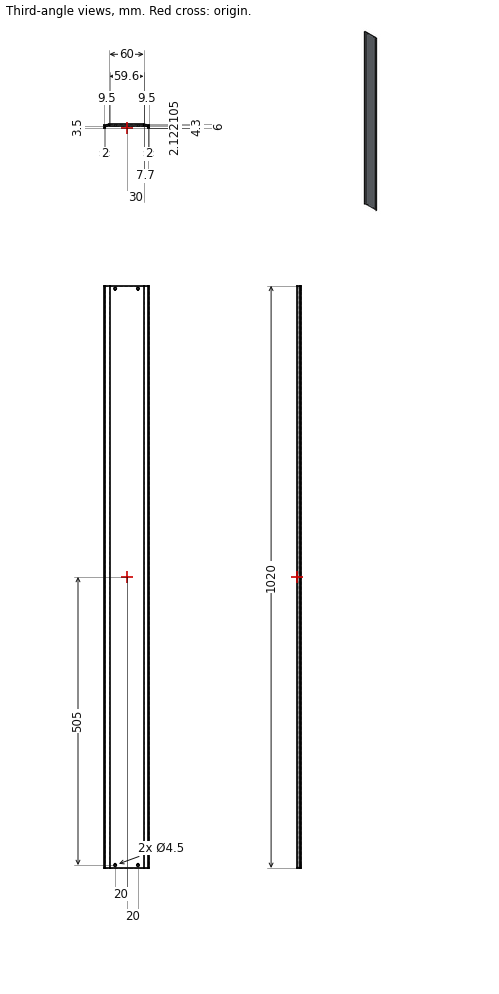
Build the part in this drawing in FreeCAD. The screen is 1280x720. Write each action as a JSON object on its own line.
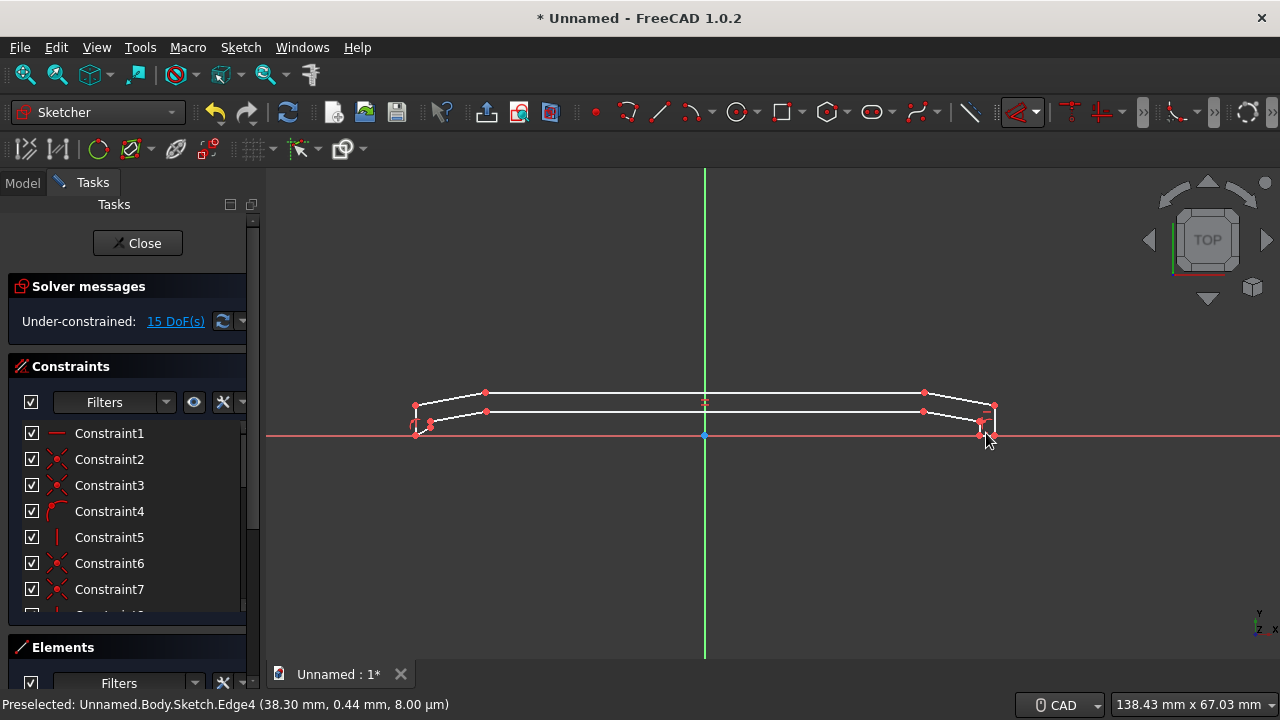
{"action": "scroll", "coordinate": [426, 430], "scroll_direction": "up", "scroll_amount": 5}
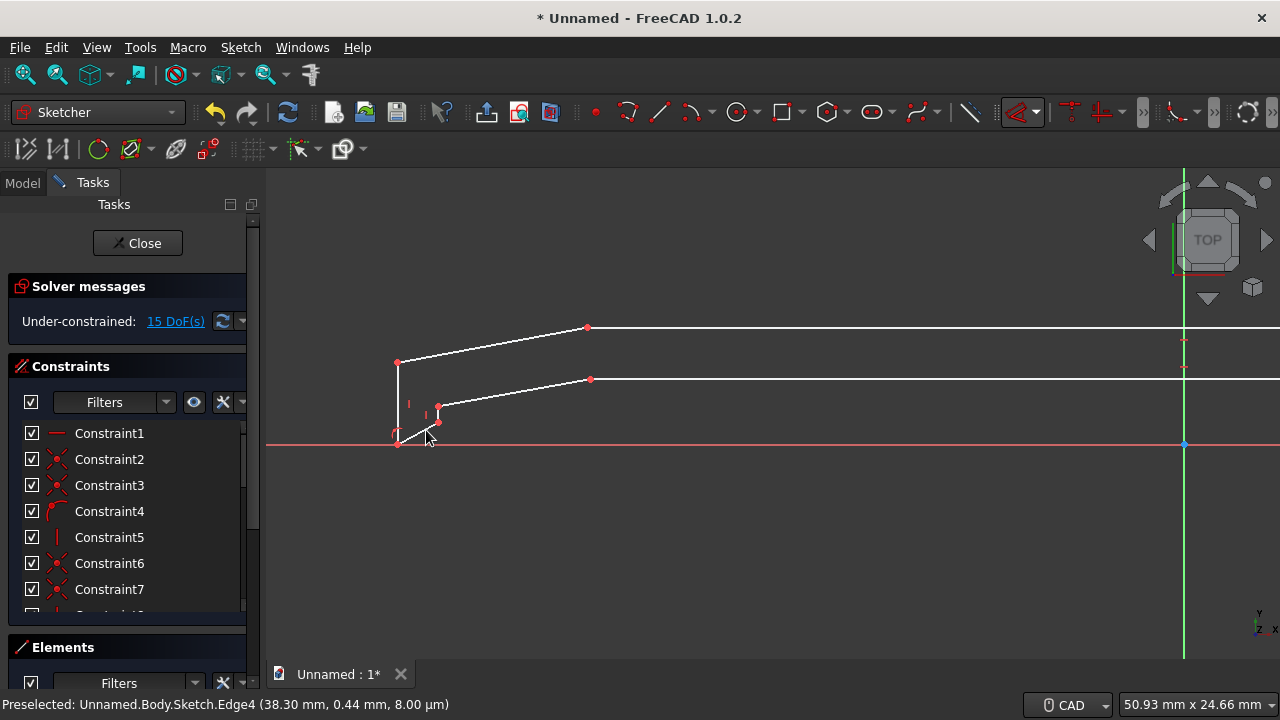
{"action": "left_click", "coordinate": [426, 429]}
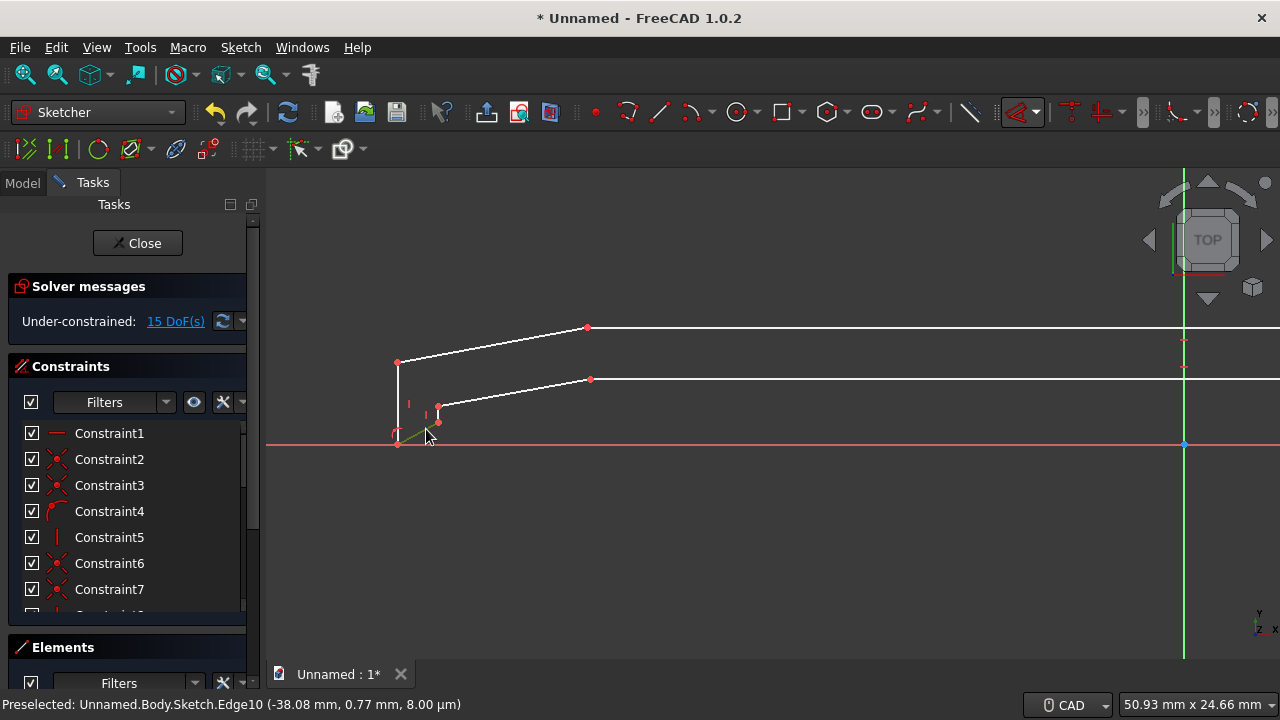
{"action": "left_click", "coordinate": [1124, 112]}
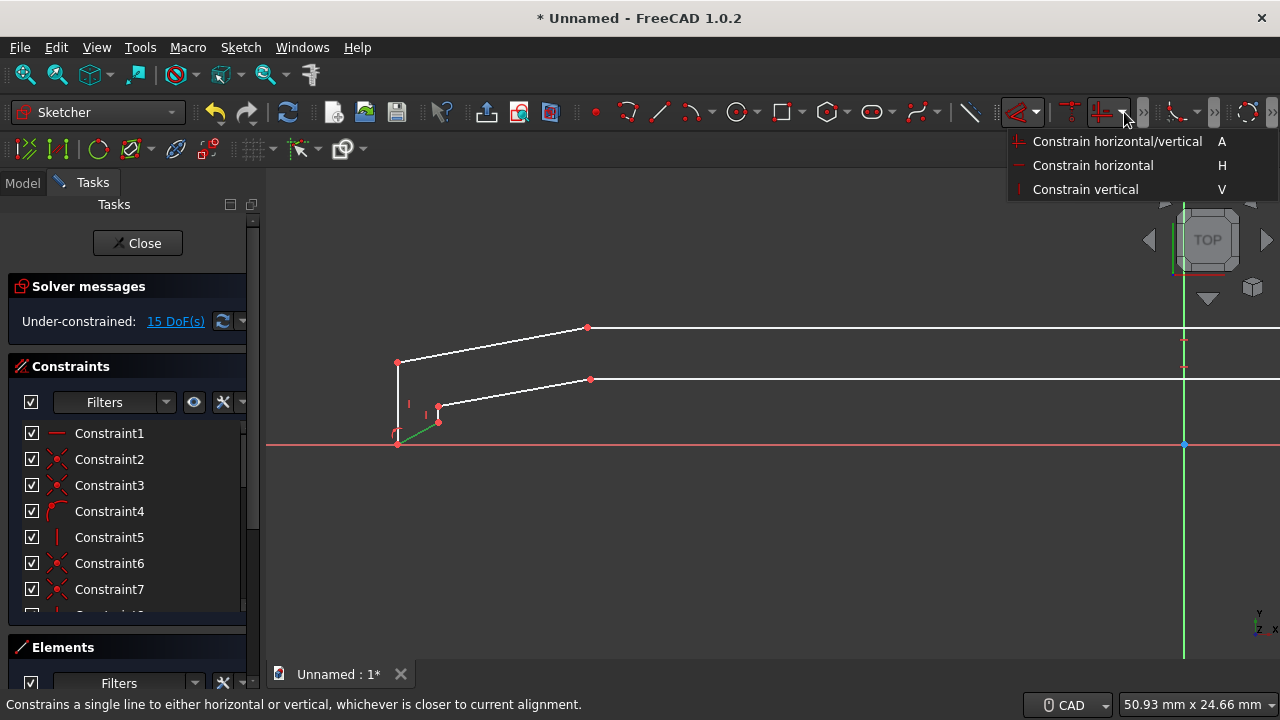
{"action": "left_click", "coordinate": [1143, 165]}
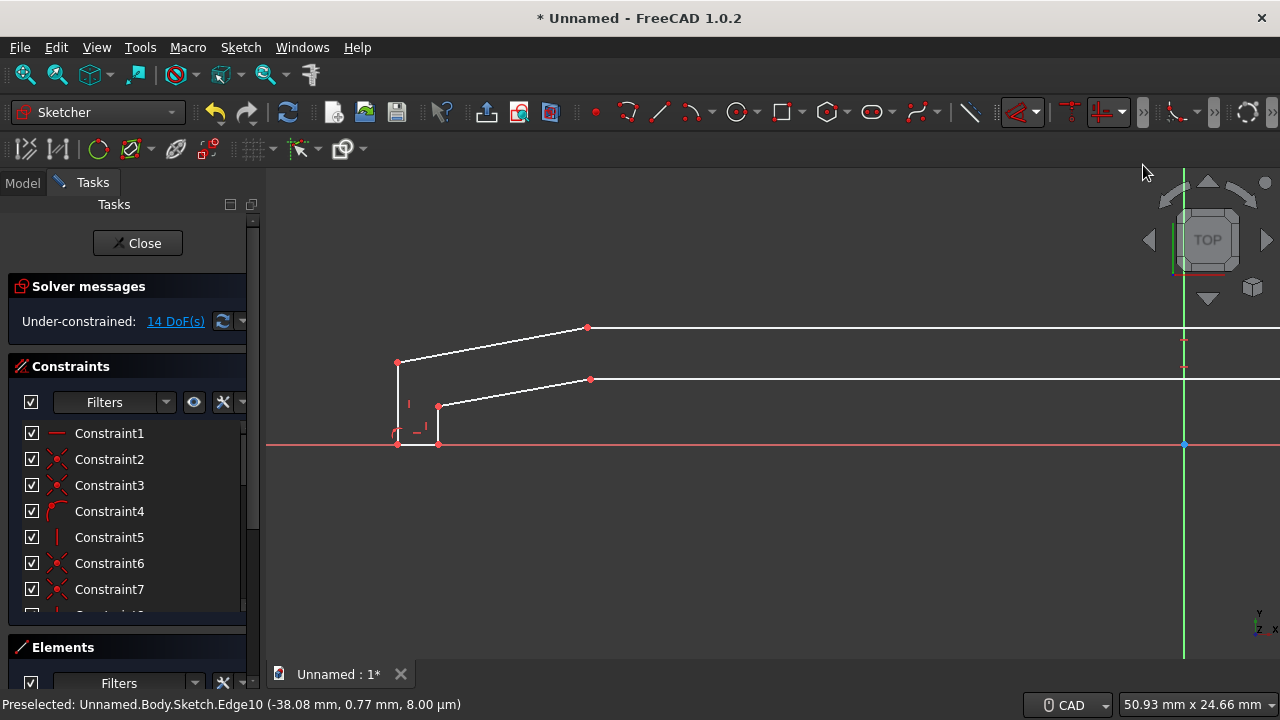
{"action": "scroll", "coordinate": [425, 430], "scroll_direction": "down", "scroll_amount": 5}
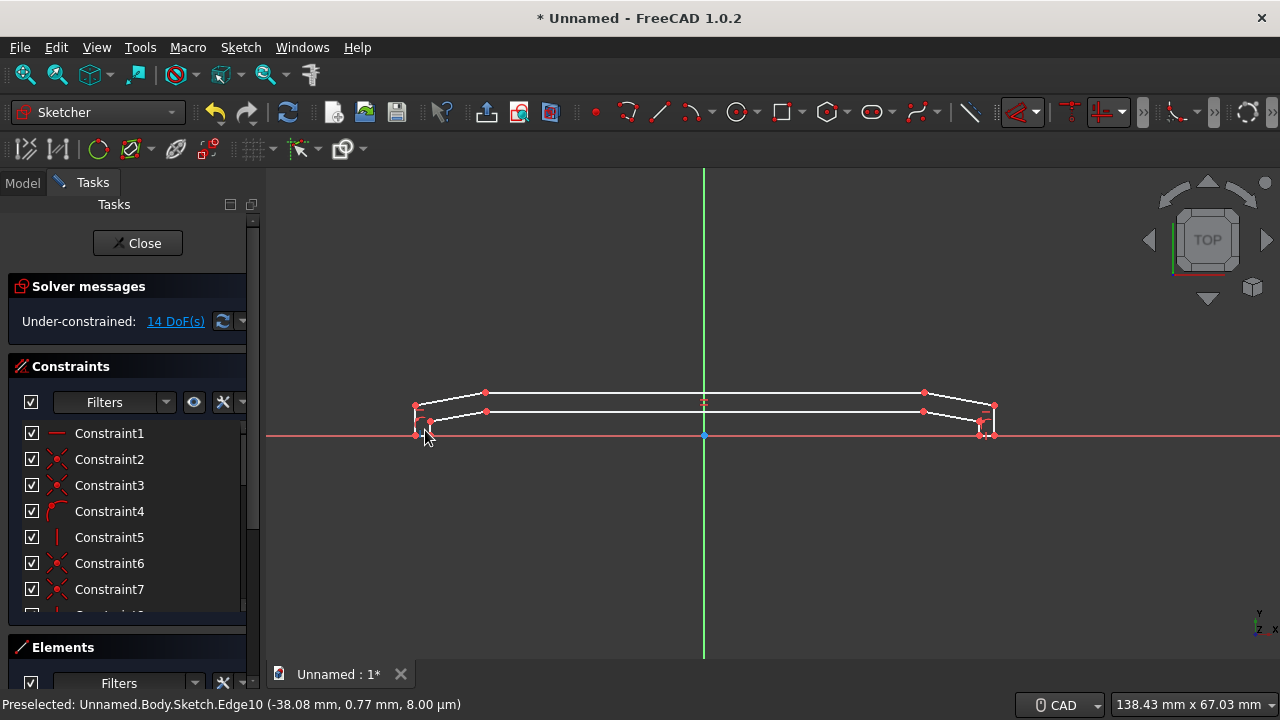
{"action": "scroll", "coordinate": [983, 436], "scroll_direction": "up", "scroll_amount": 6}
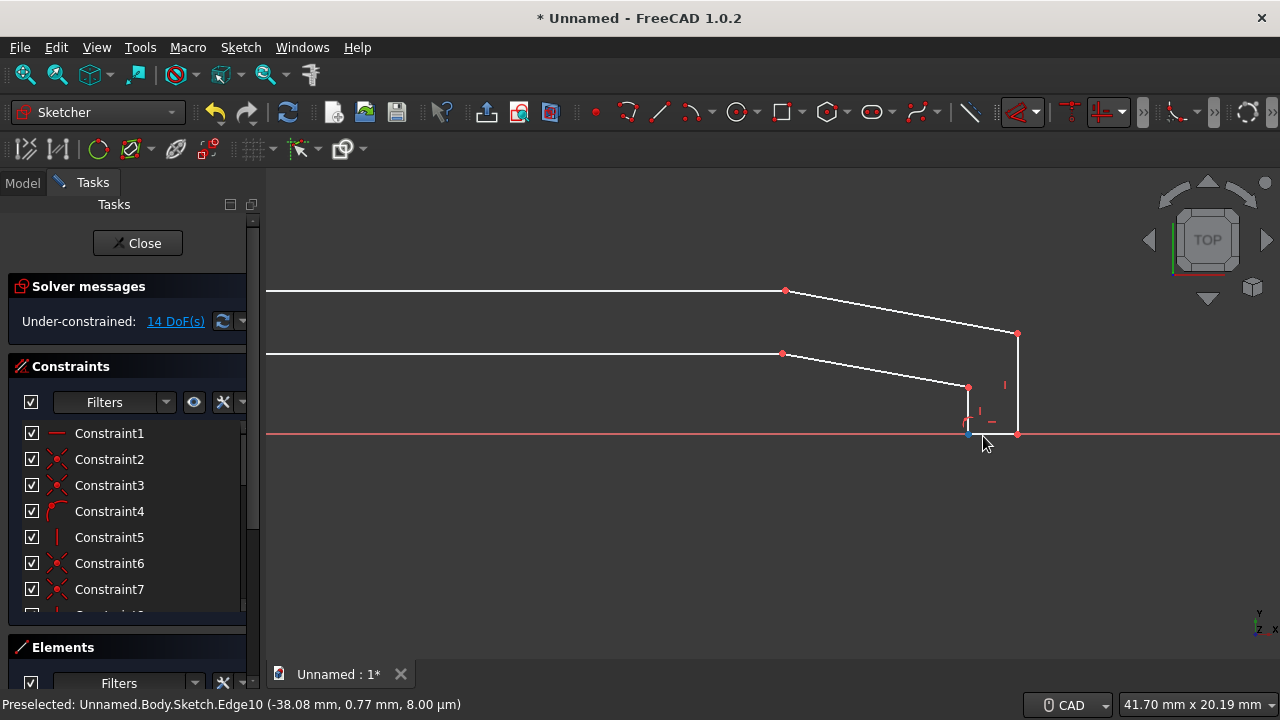
{"action": "left_click", "coordinate": [983, 434]}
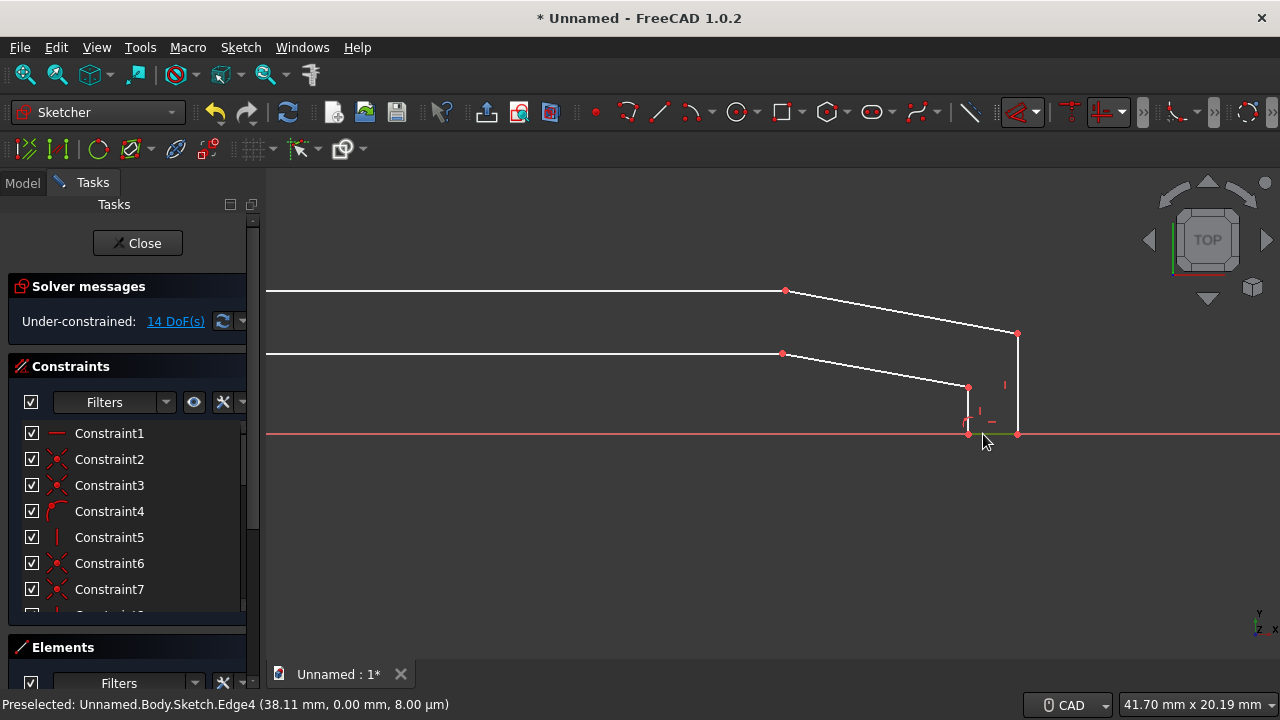
{"action": "key", "text": "l"}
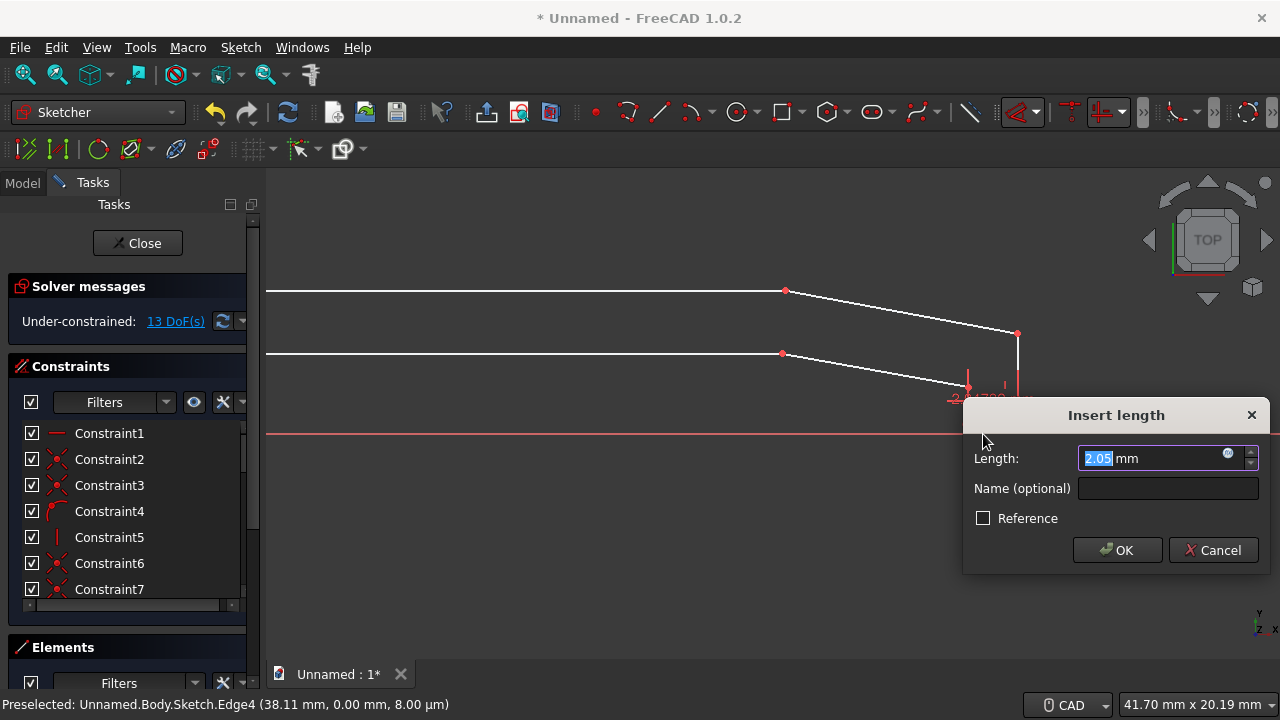
{"action": "type", "text": "2"}
{"action": "key", "text": "Return"}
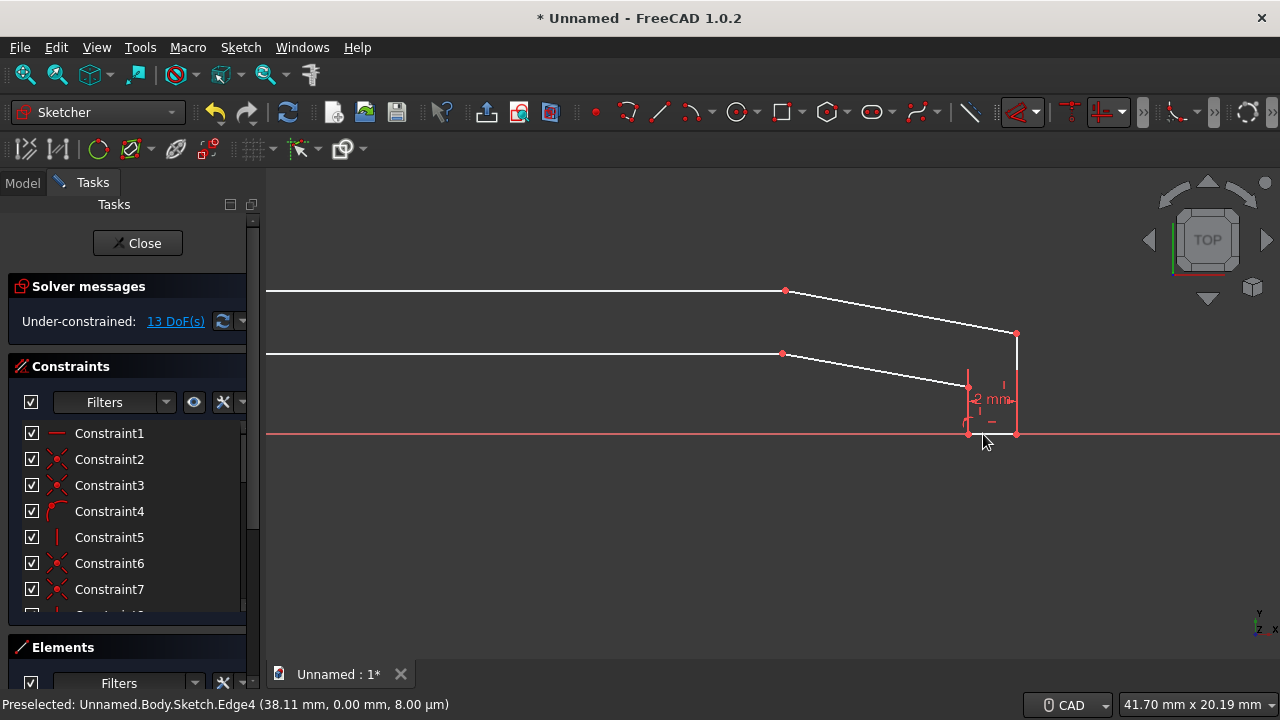
{"action": "scroll", "coordinate": [984, 436], "scroll_direction": "down", "scroll_amount": 6}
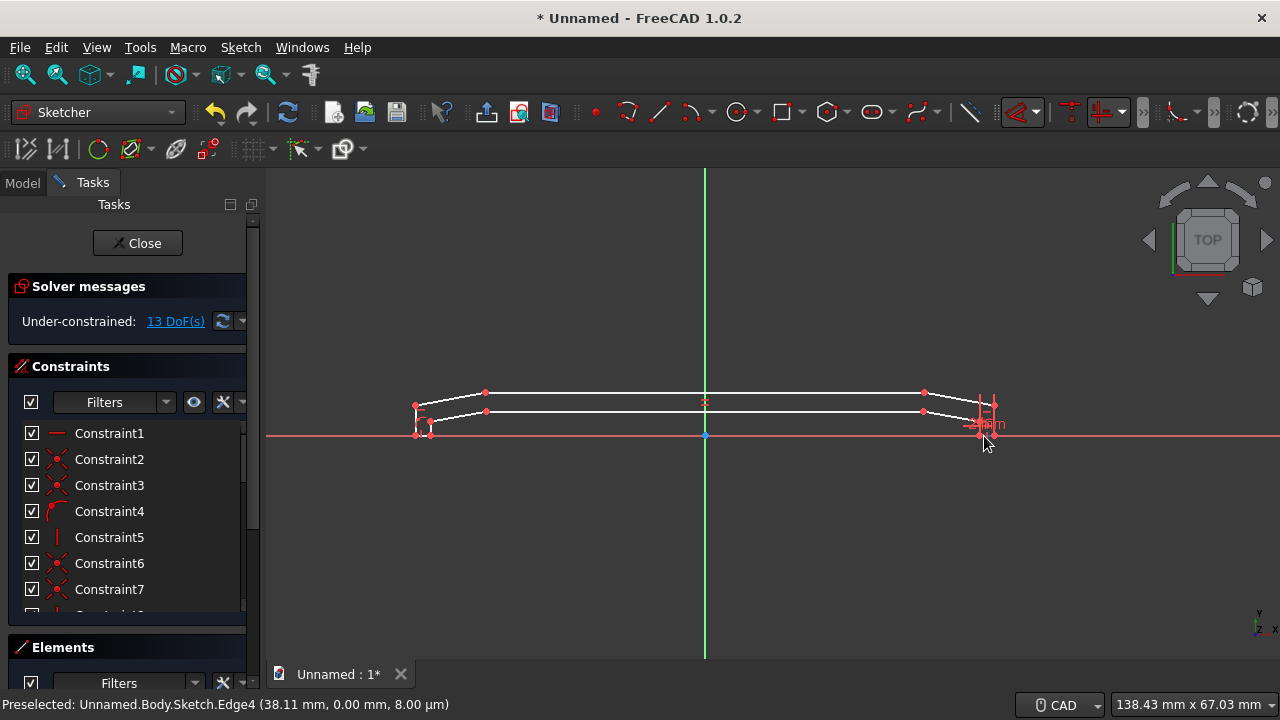
{"action": "scroll", "coordinate": [420, 436], "scroll_direction": "up", "scroll_amount": 6}